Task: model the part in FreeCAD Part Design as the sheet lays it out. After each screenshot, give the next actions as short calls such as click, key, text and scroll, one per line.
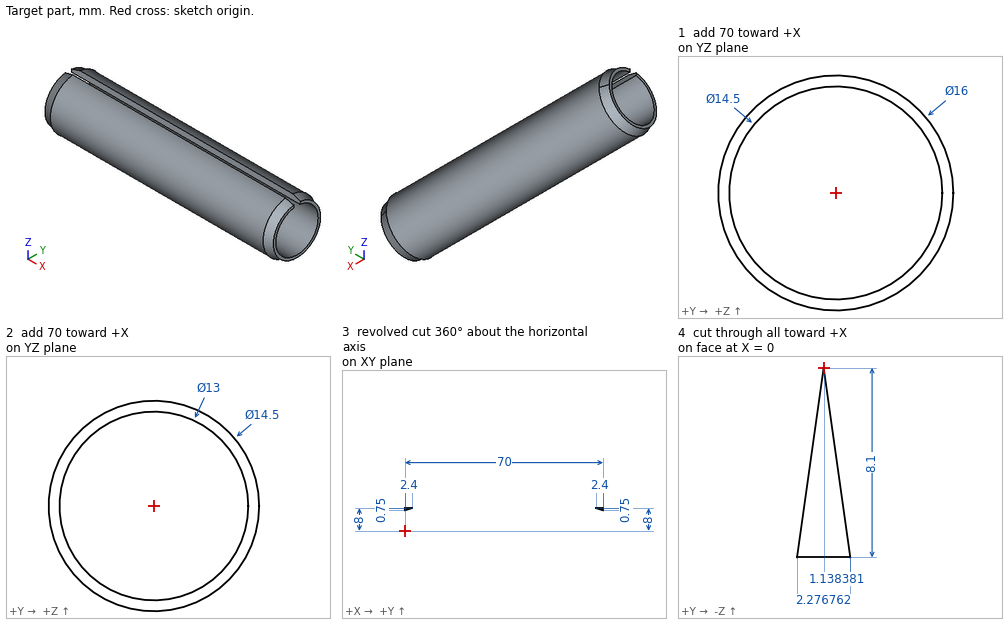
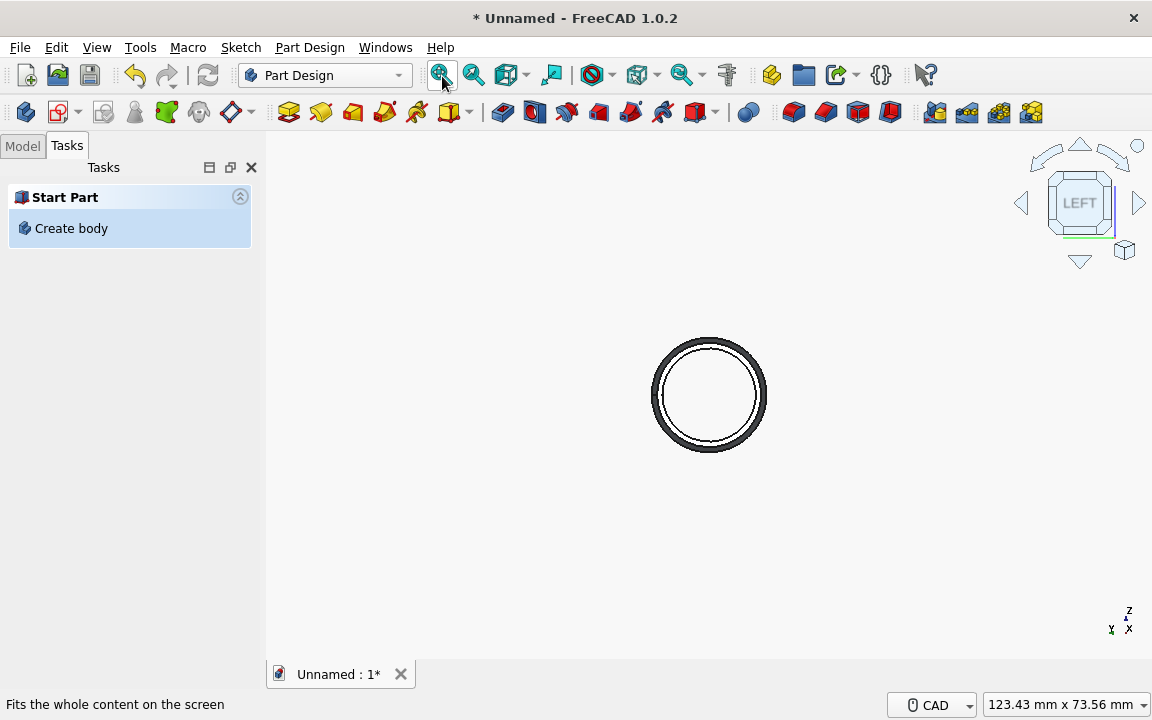
scroll(724, 439, up, 15)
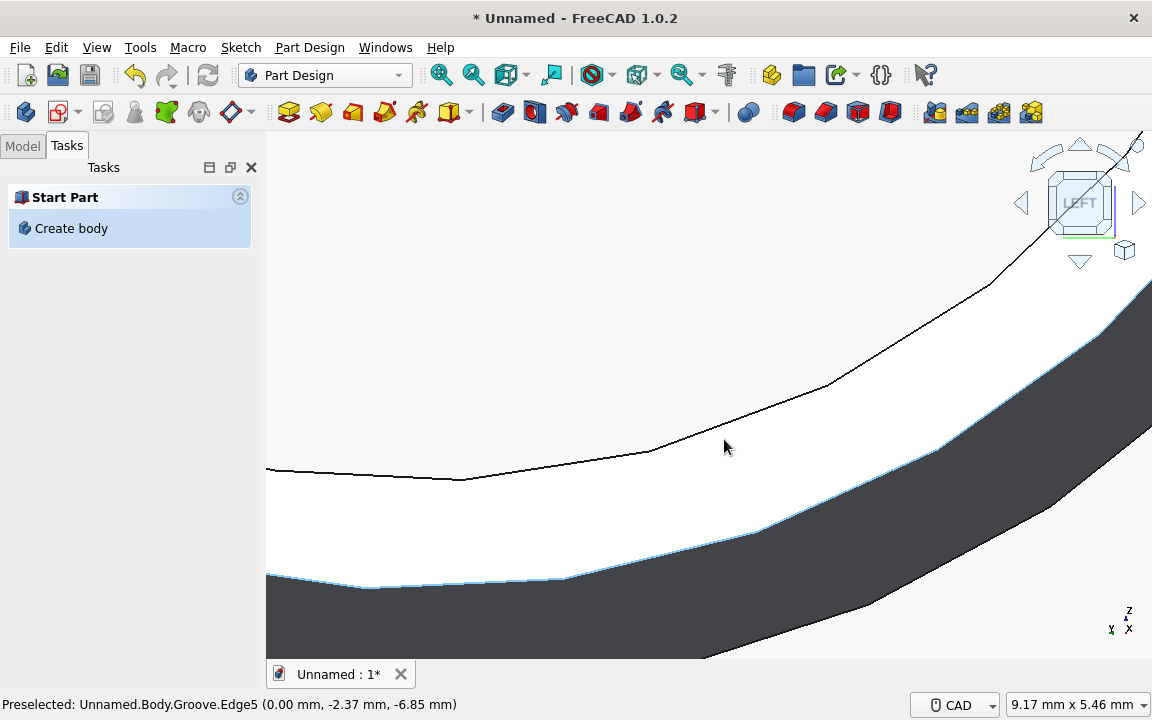
click(714, 439)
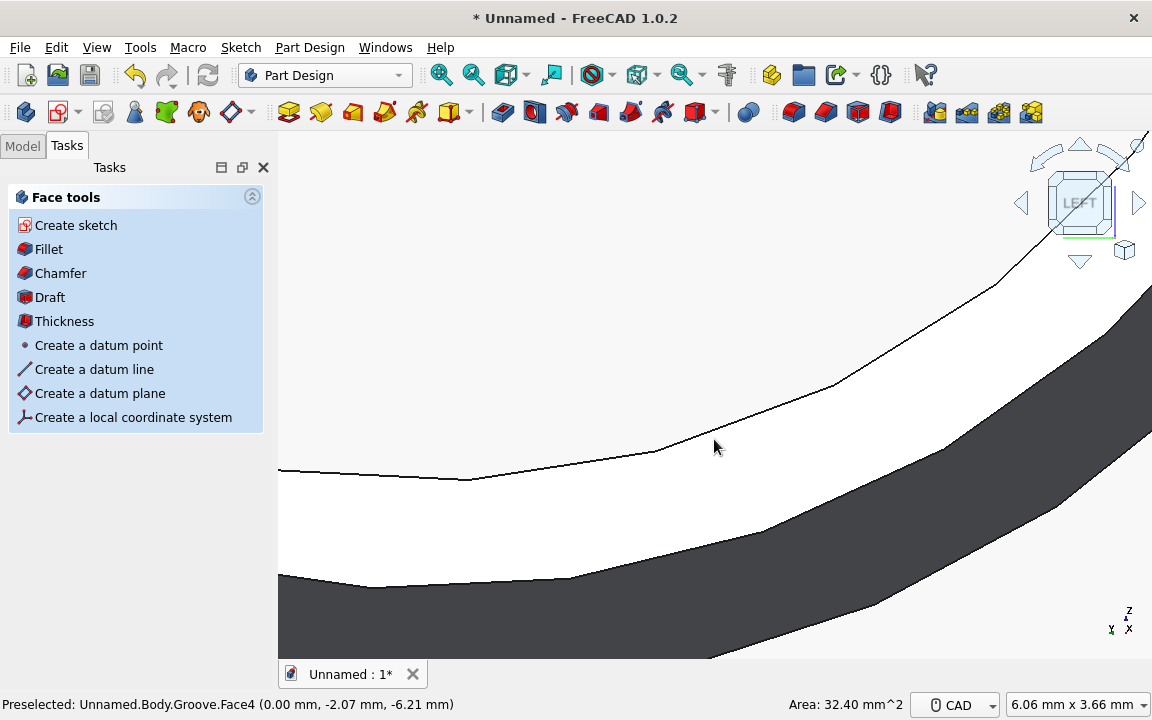
click(58, 112)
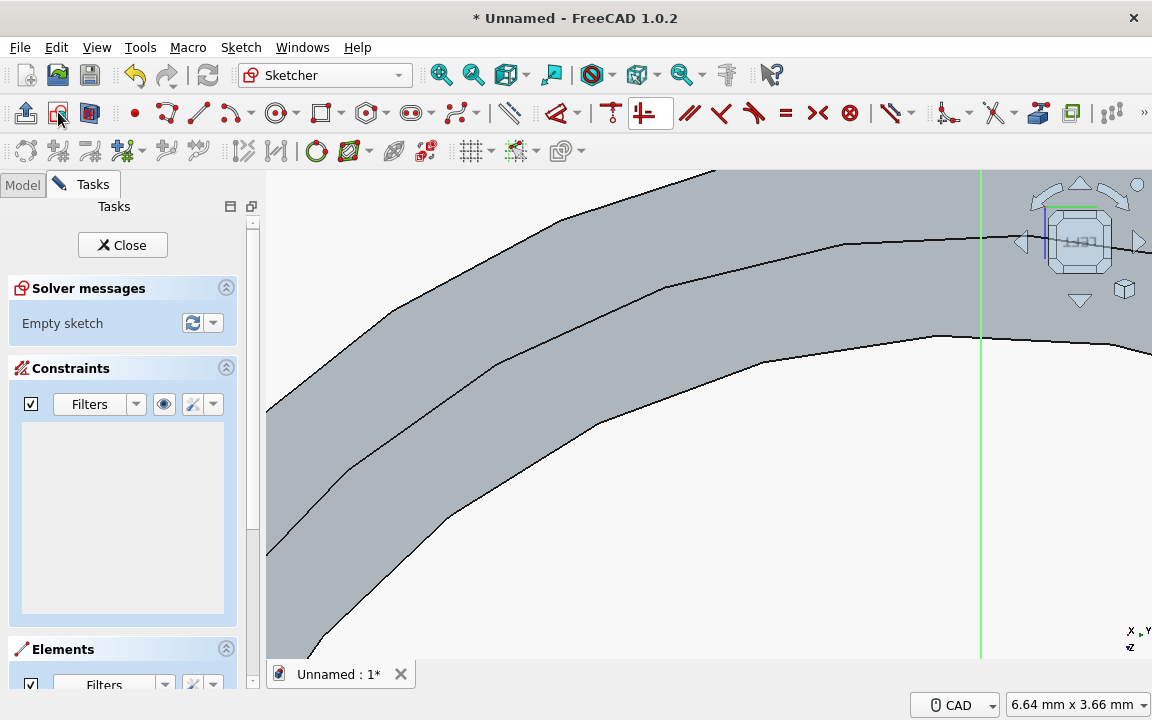
scroll(573, 198, down, 9)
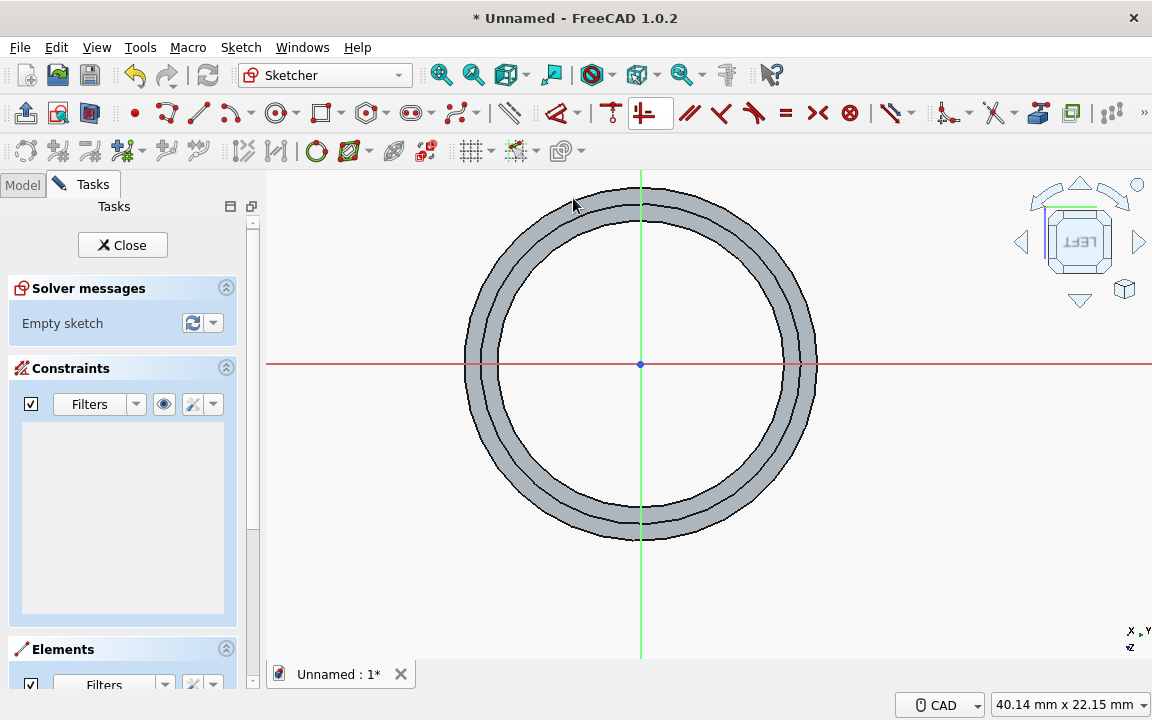
scroll(641, 501, up, 3)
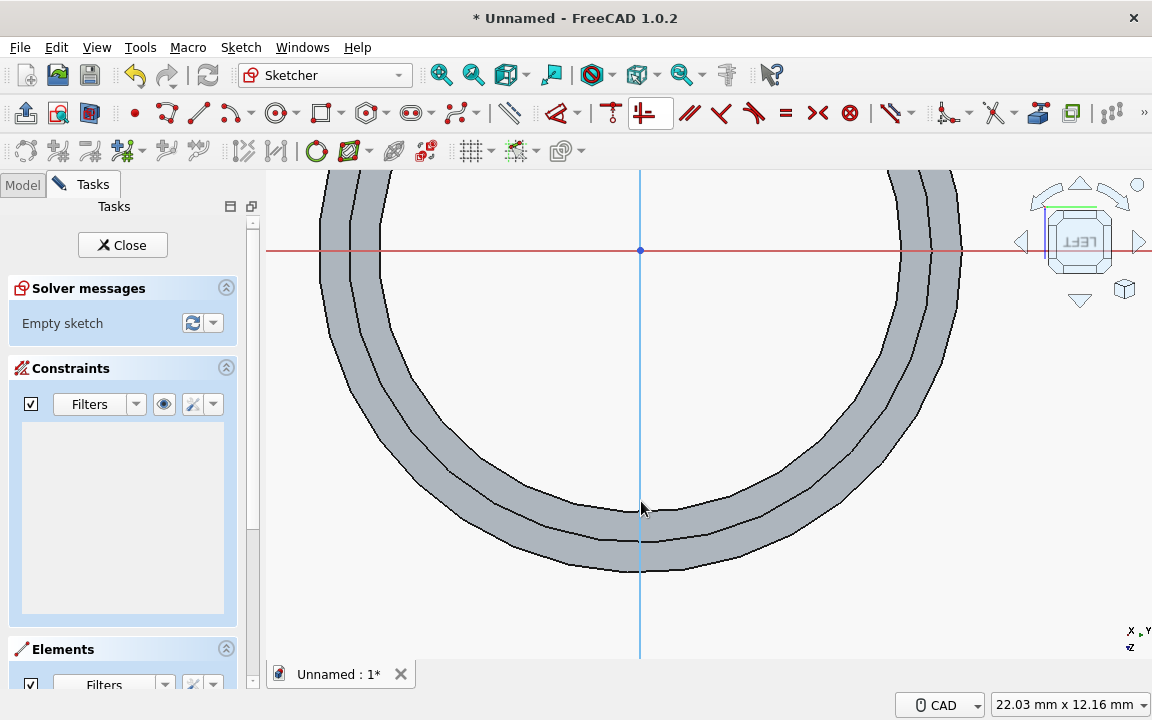
click(168, 114)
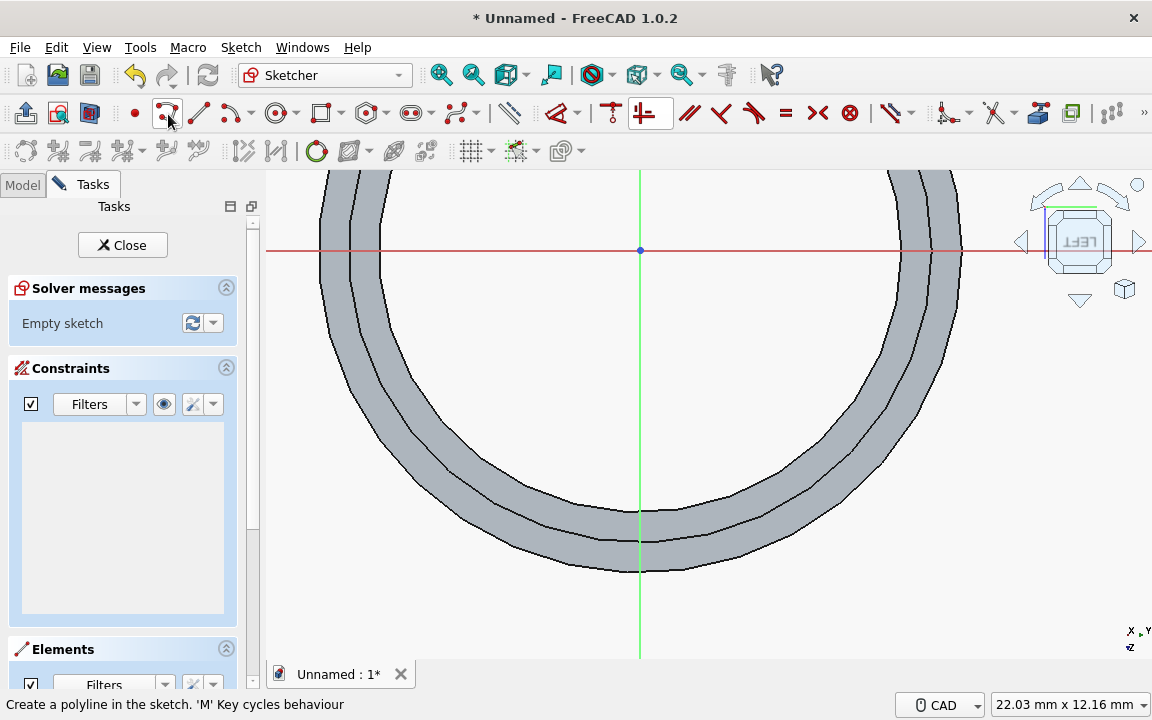
click(640, 251)
click(686, 577)
click(594, 577)
click(640, 251)
key(Escape)
key(Escape)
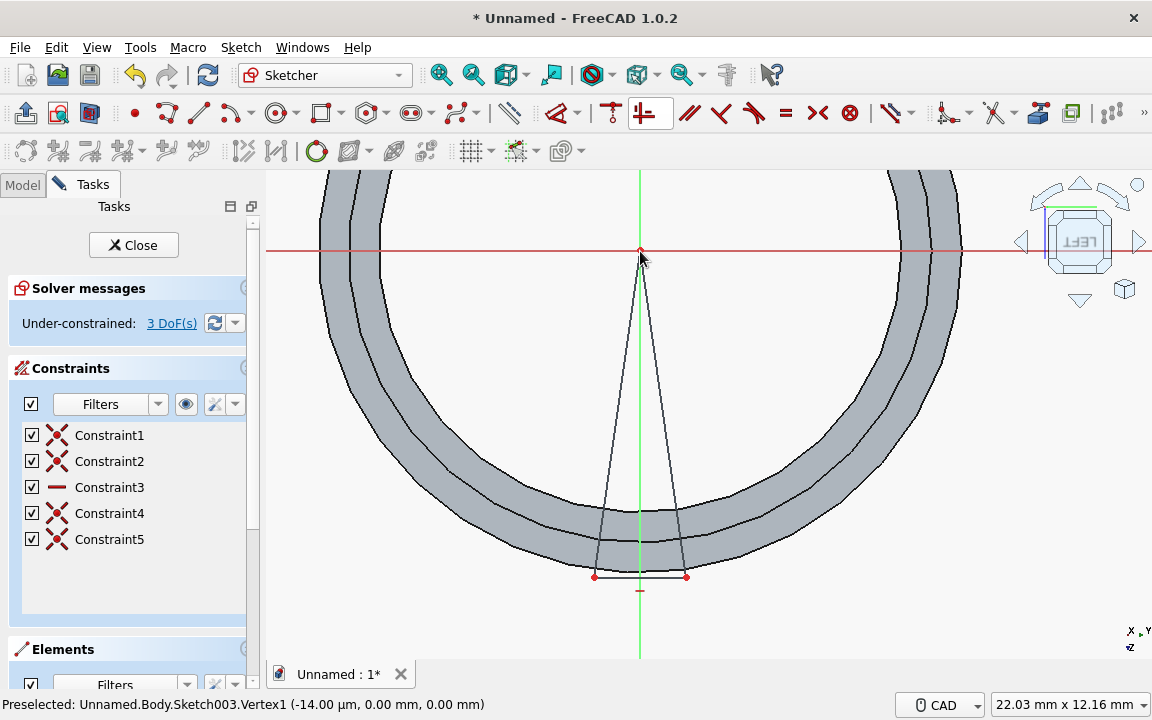
click(556, 114)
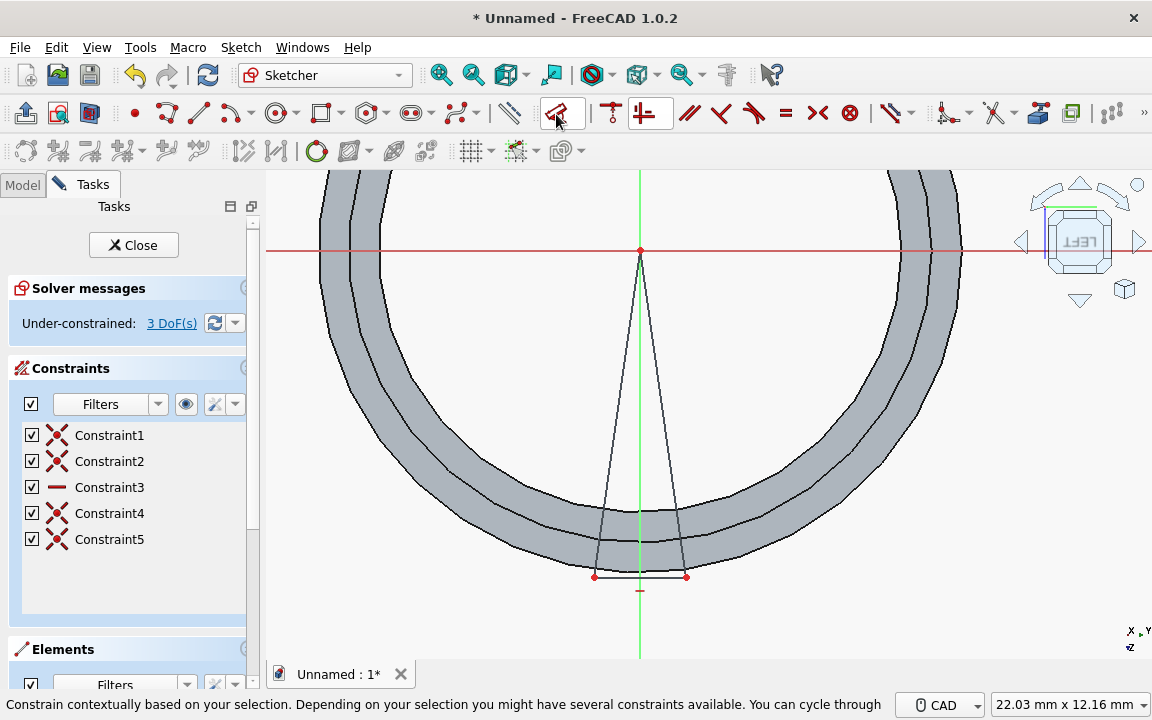
click(686, 578)
click(720, 414)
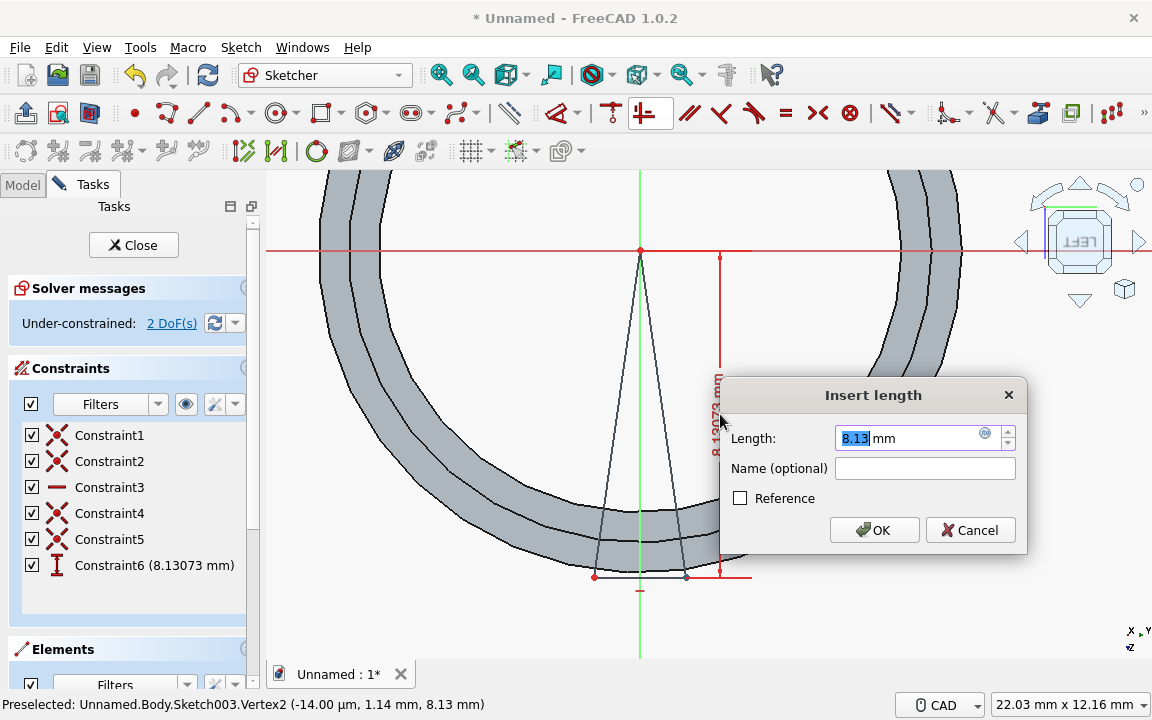
text(8.1)
key(Return)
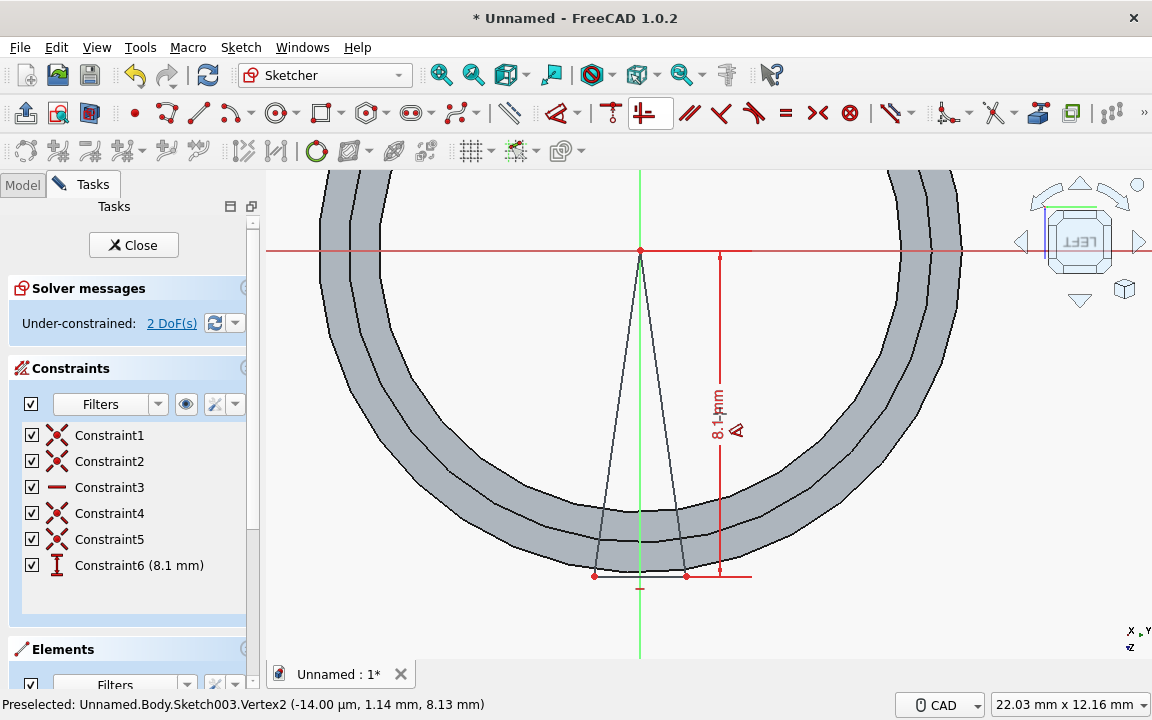
click(658, 577)
click(619, 611)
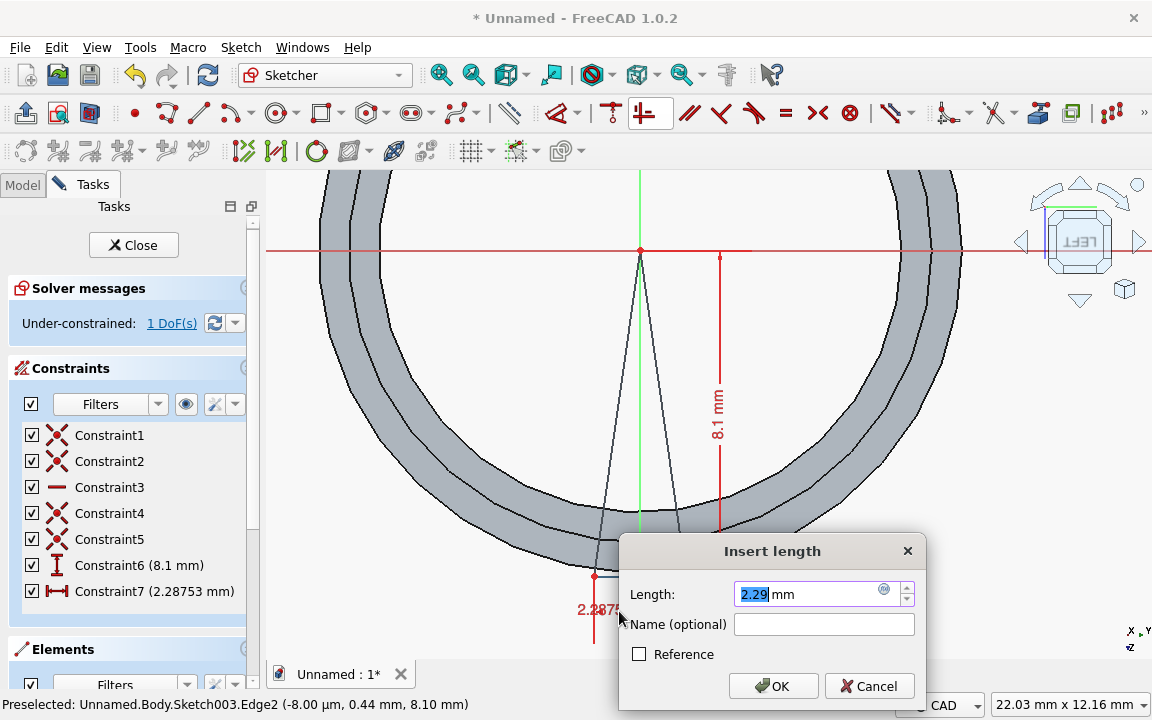
text(2.276762)
key(Return)